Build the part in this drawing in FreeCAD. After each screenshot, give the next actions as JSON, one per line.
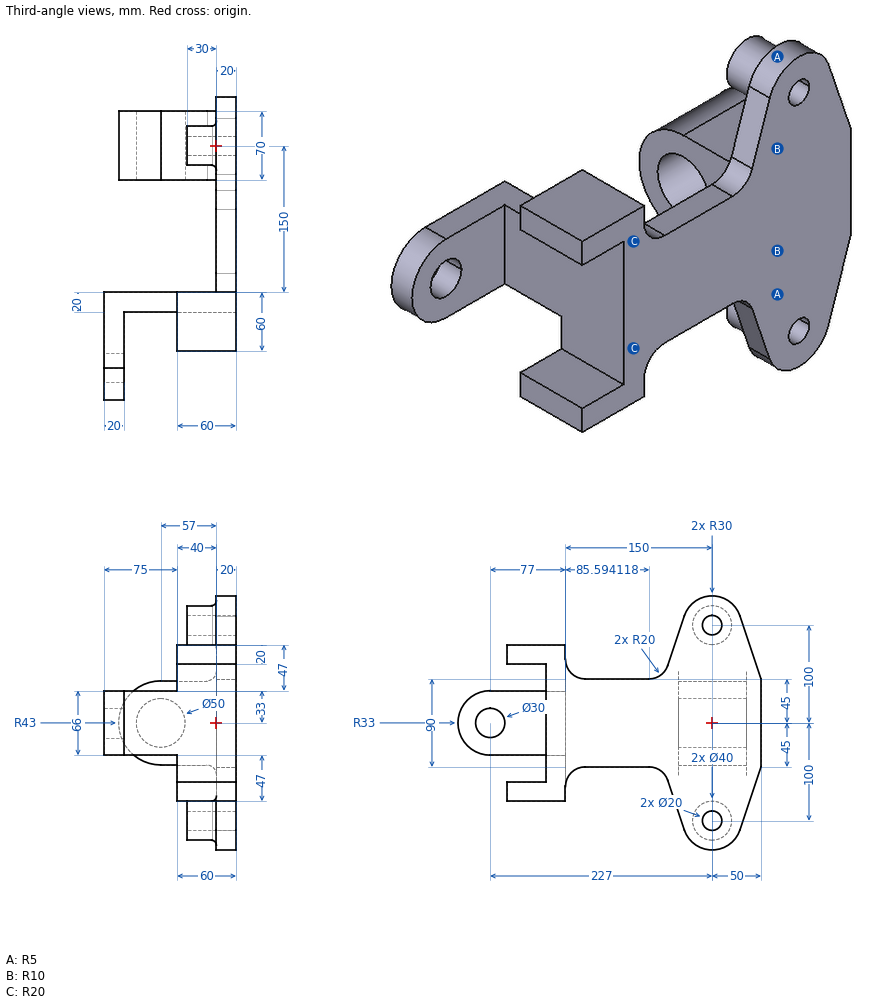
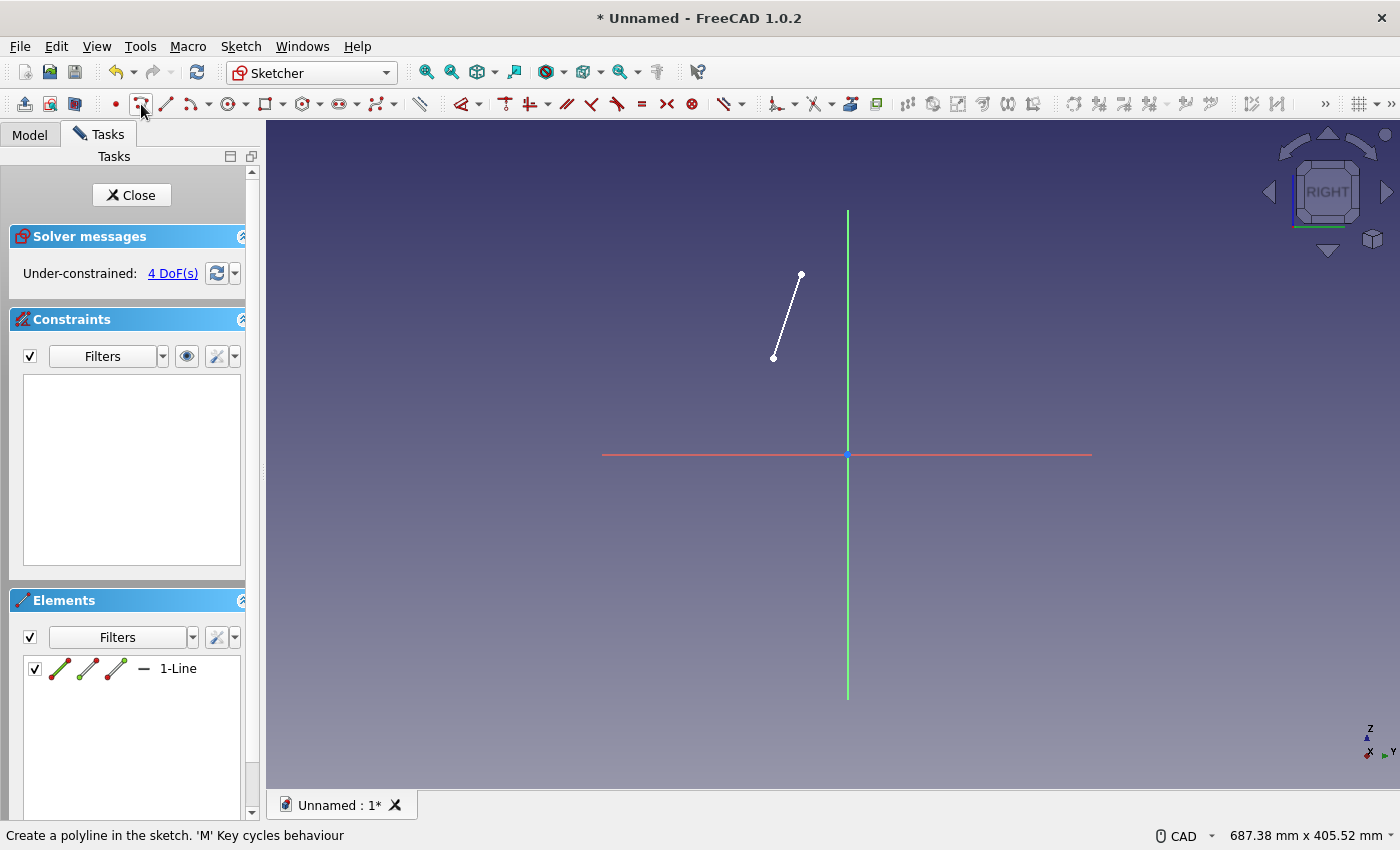
{"action": "left_click", "coordinate": [741, 380]}
{"action": "left_click", "coordinate": [600, 380]}
{"action": "left_click", "coordinate": [600, 529]}
{"action": "left_click", "coordinate": [741, 529]}
{"action": "right_click", "coordinate": [741, 529]}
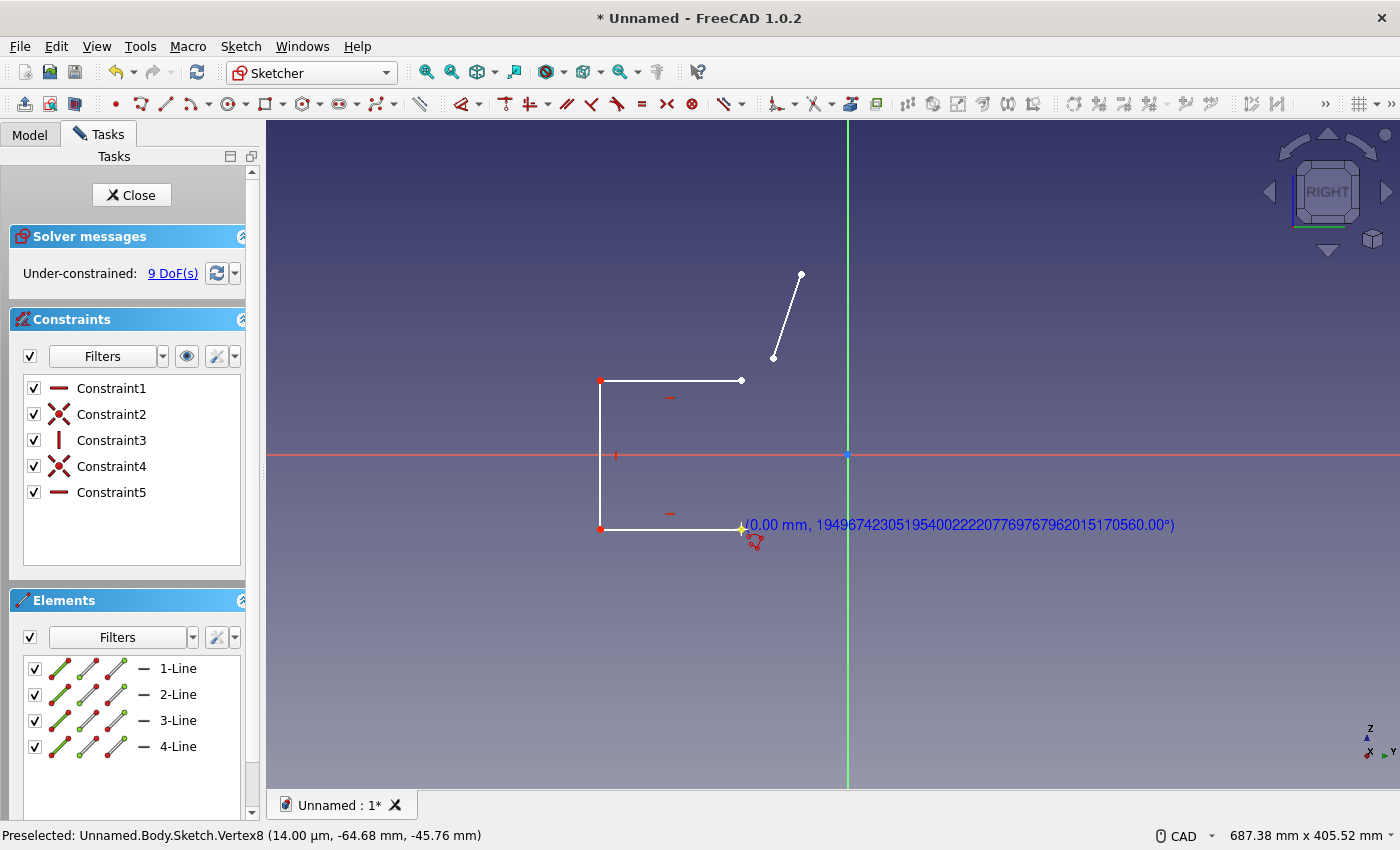
{"action": "left_click", "coordinate": [166, 104]}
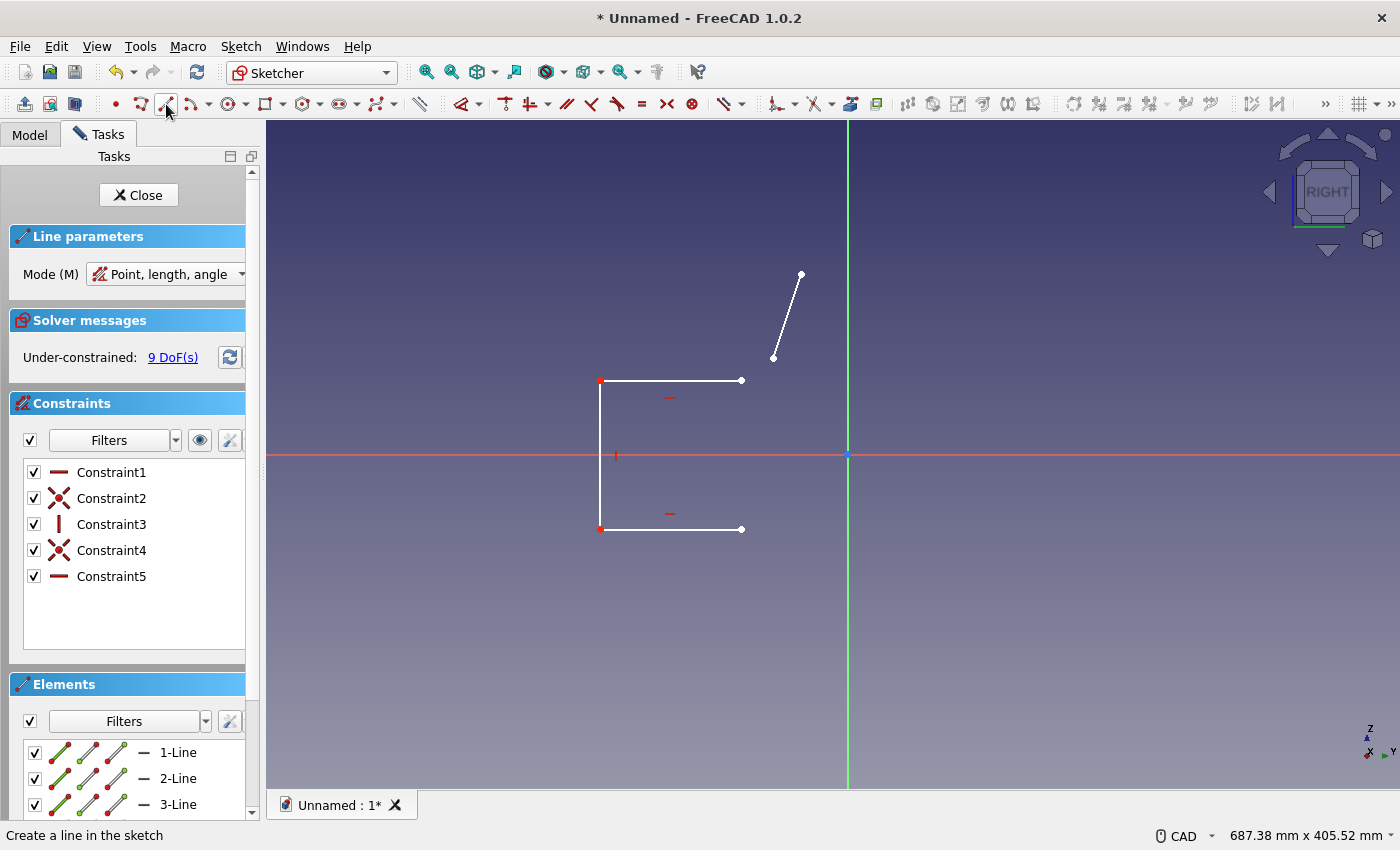
{"action": "left_click", "coordinate": [773, 551]}
{"action": "left_click", "coordinate": [801, 635]}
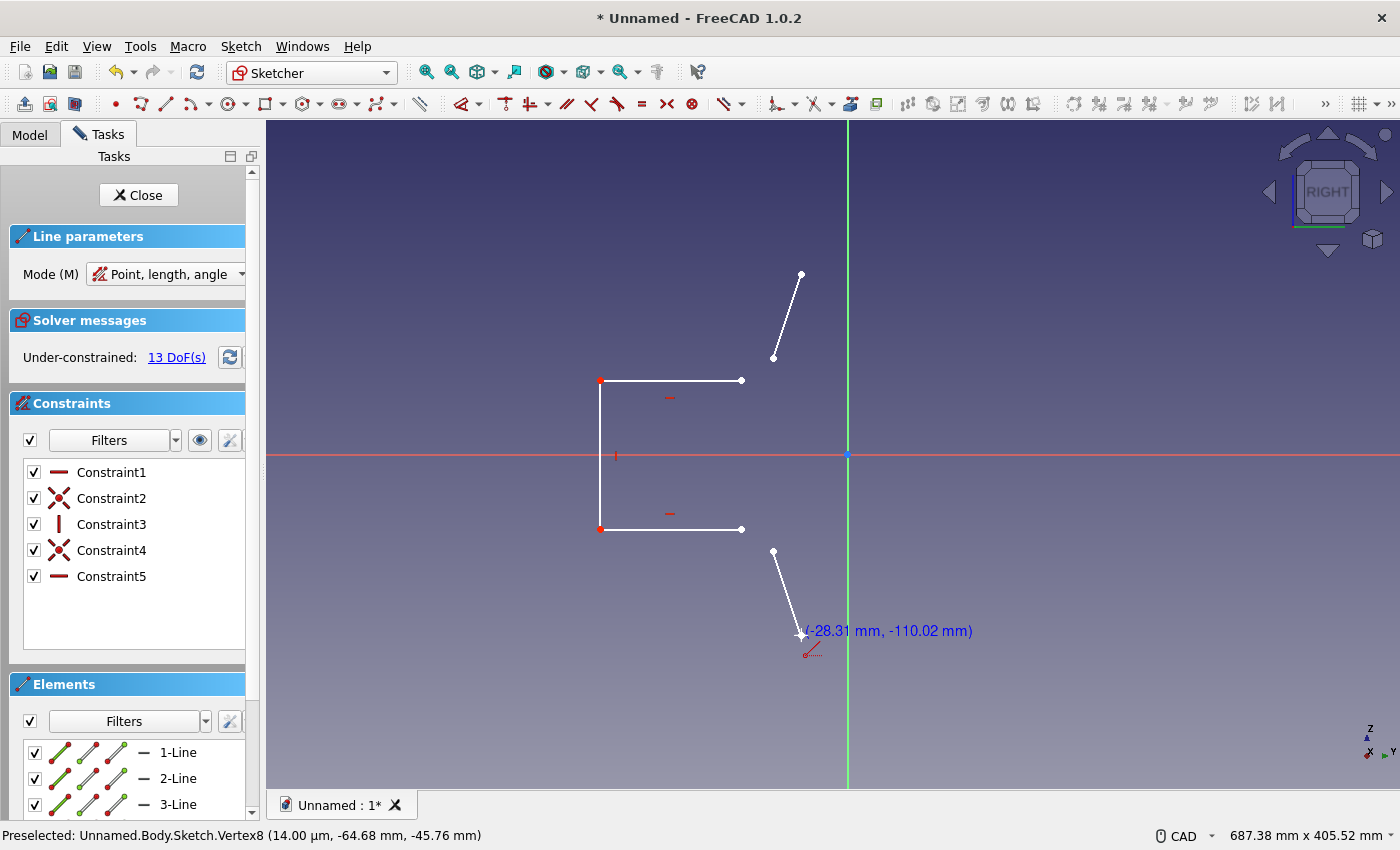
{"action": "left_click", "coordinate": [141, 104]}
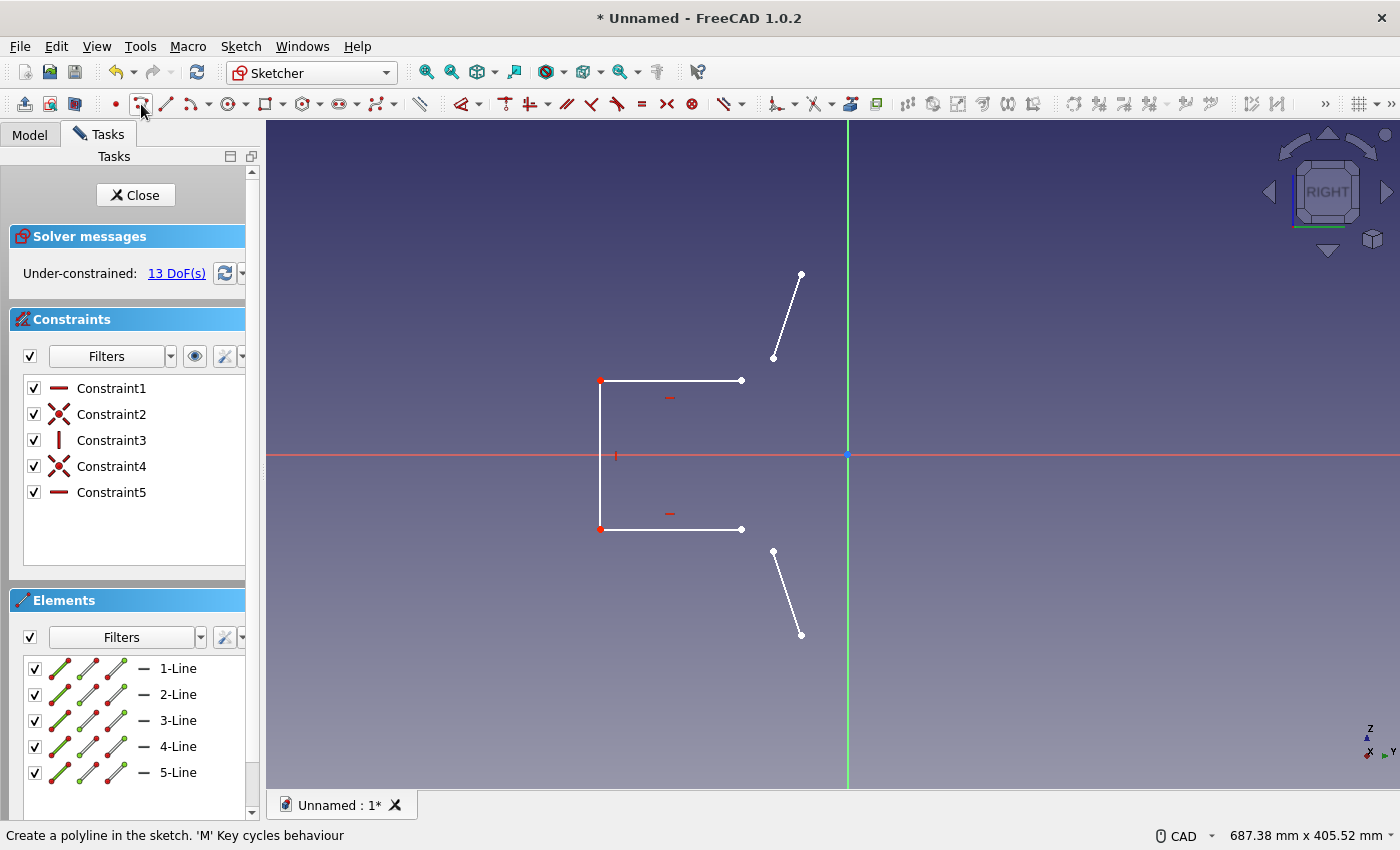
{"action": "left_click", "coordinate": [895, 635]}
{"action": "left_click", "coordinate": [930, 529]}
{"action": "left_click", "coordinate": [930, 380]}
{"action": "left_click", "coordinate": [895, 274]}
{"action": "right_click", "coordinate": [895, 274]}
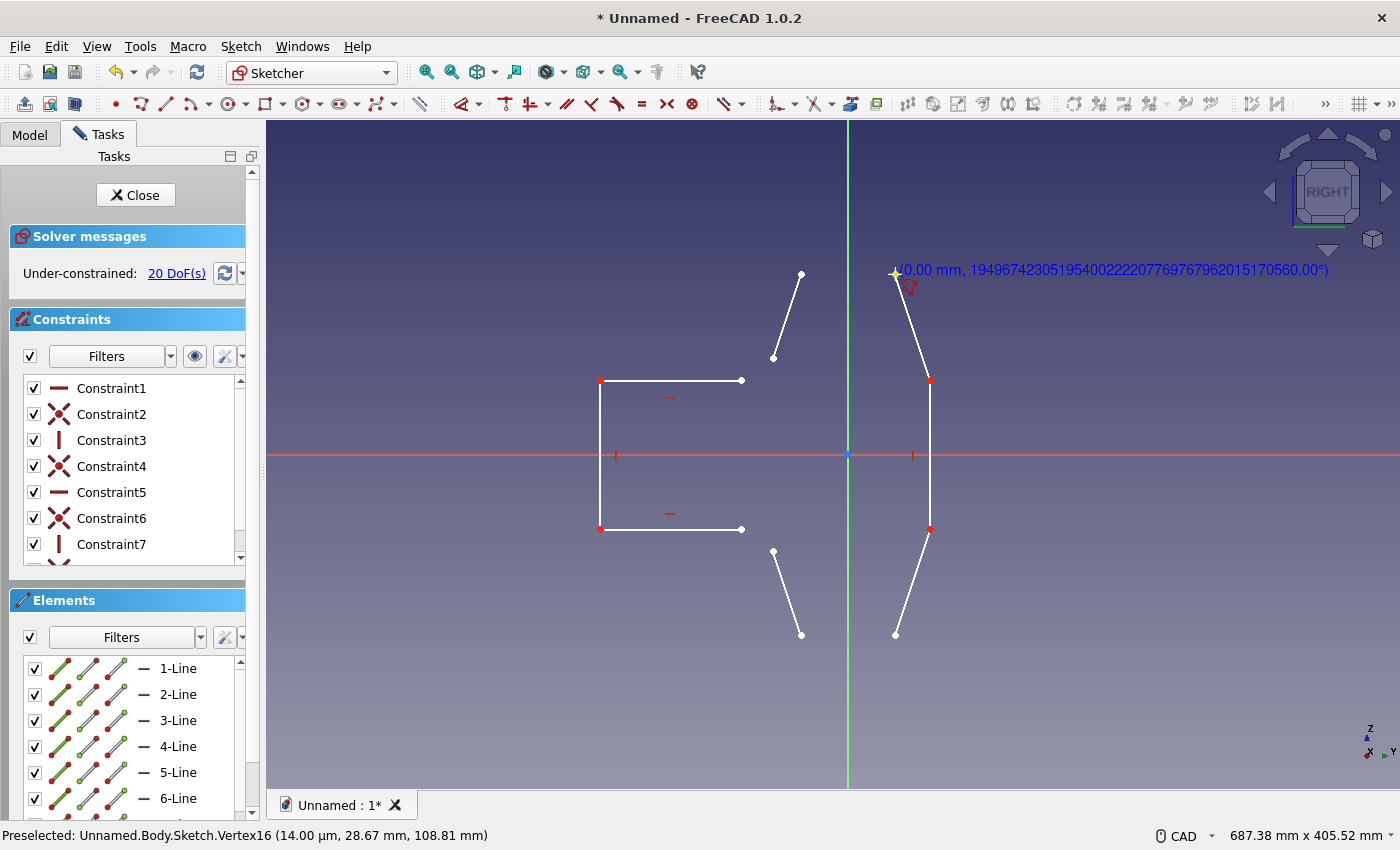
{"action": "key", "text": "g 3 a"}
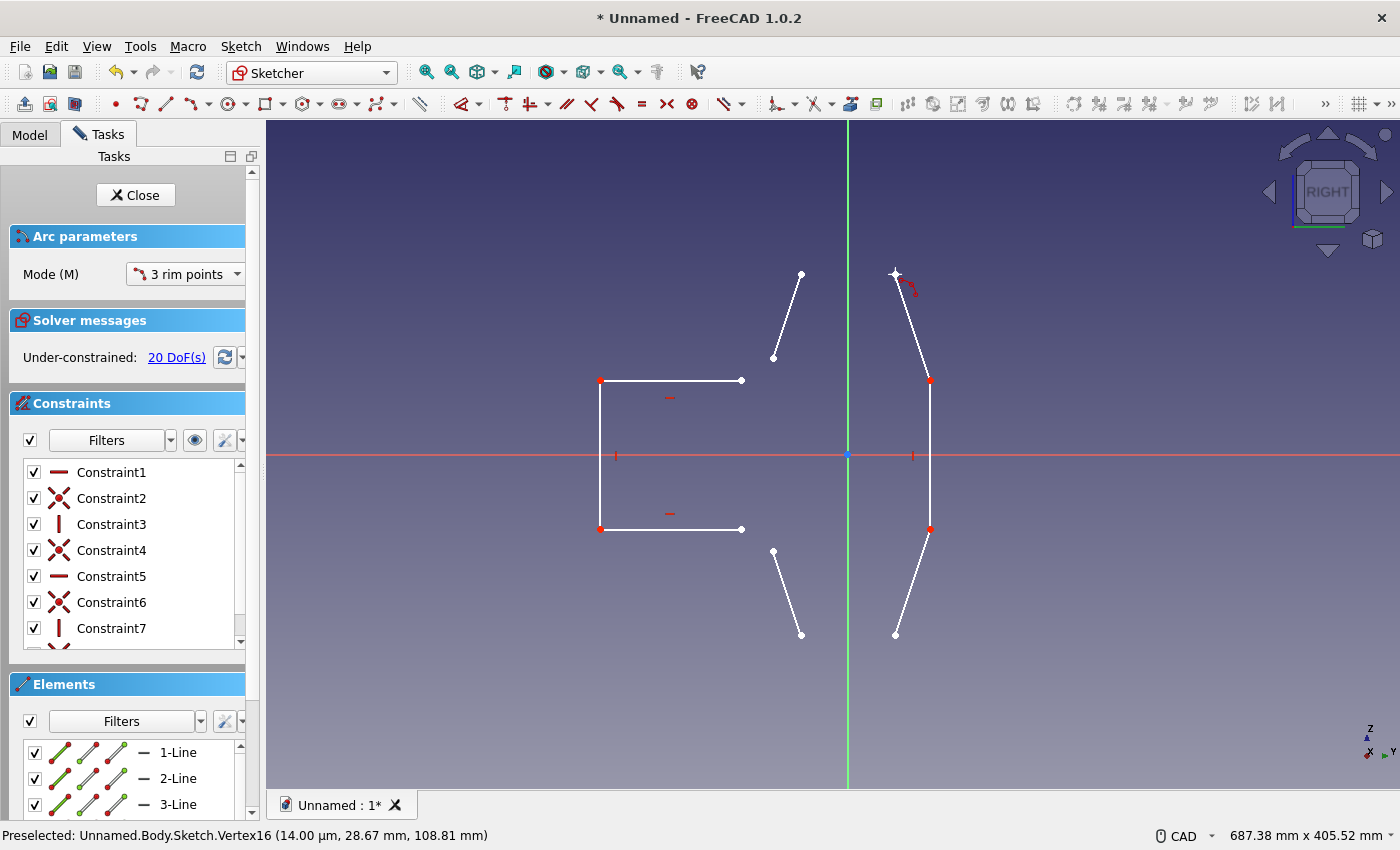
{"action": "left_click", "coordinate": [773, 359]}
{"action": "left_click", "coordinate": [741, 381]}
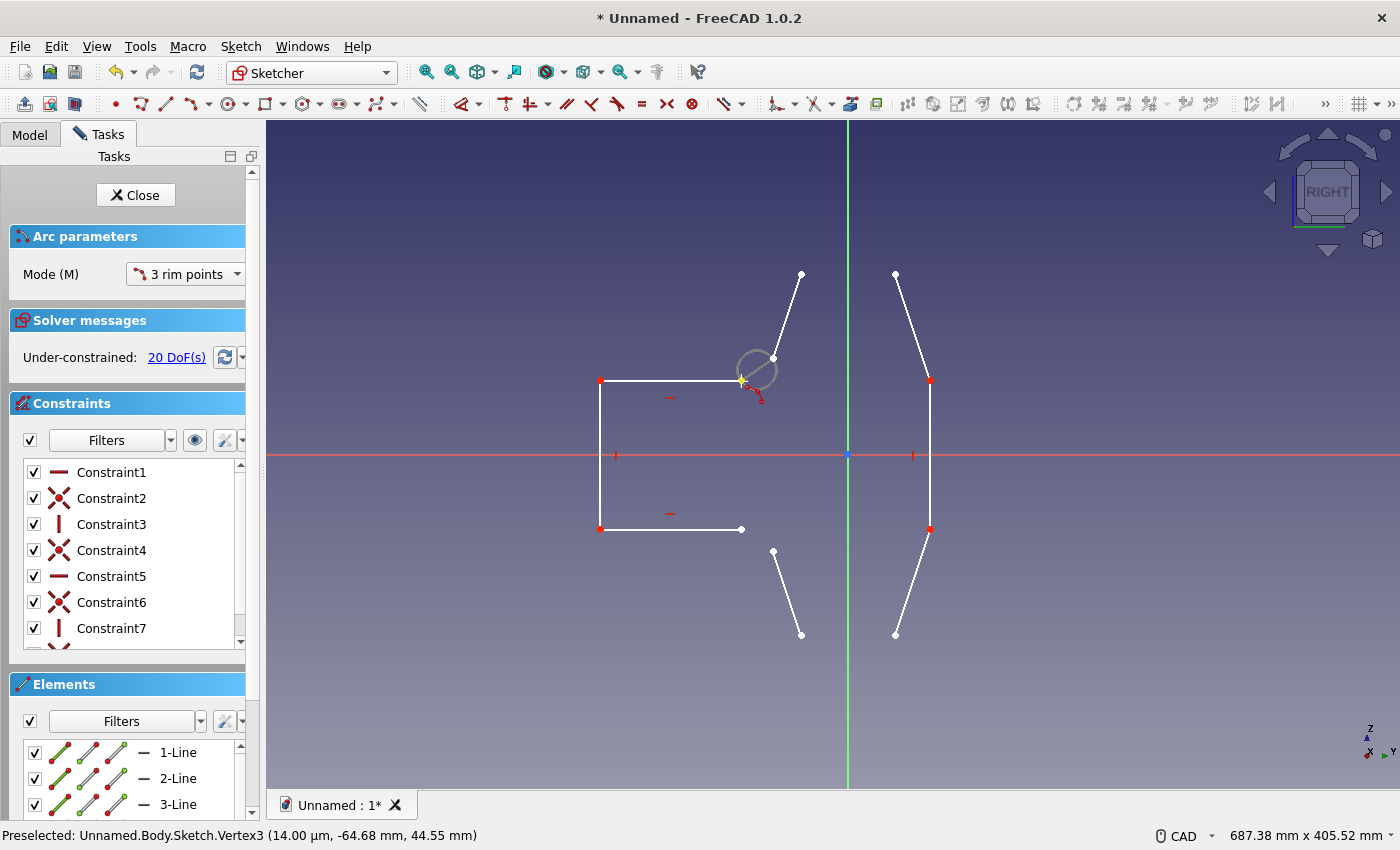
{"action": "scroll", "coordinate": [761, 374], "scroll_direction": "up", "scroll_amount": 5}